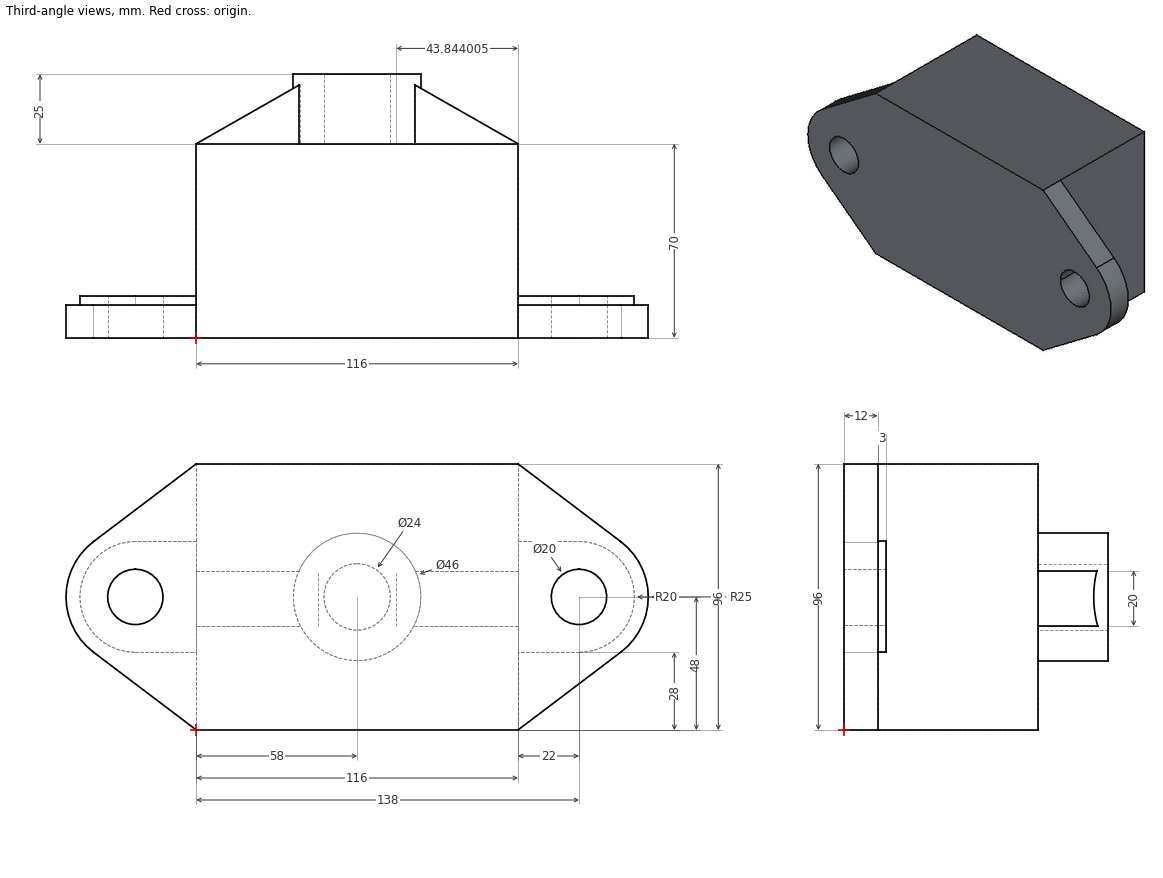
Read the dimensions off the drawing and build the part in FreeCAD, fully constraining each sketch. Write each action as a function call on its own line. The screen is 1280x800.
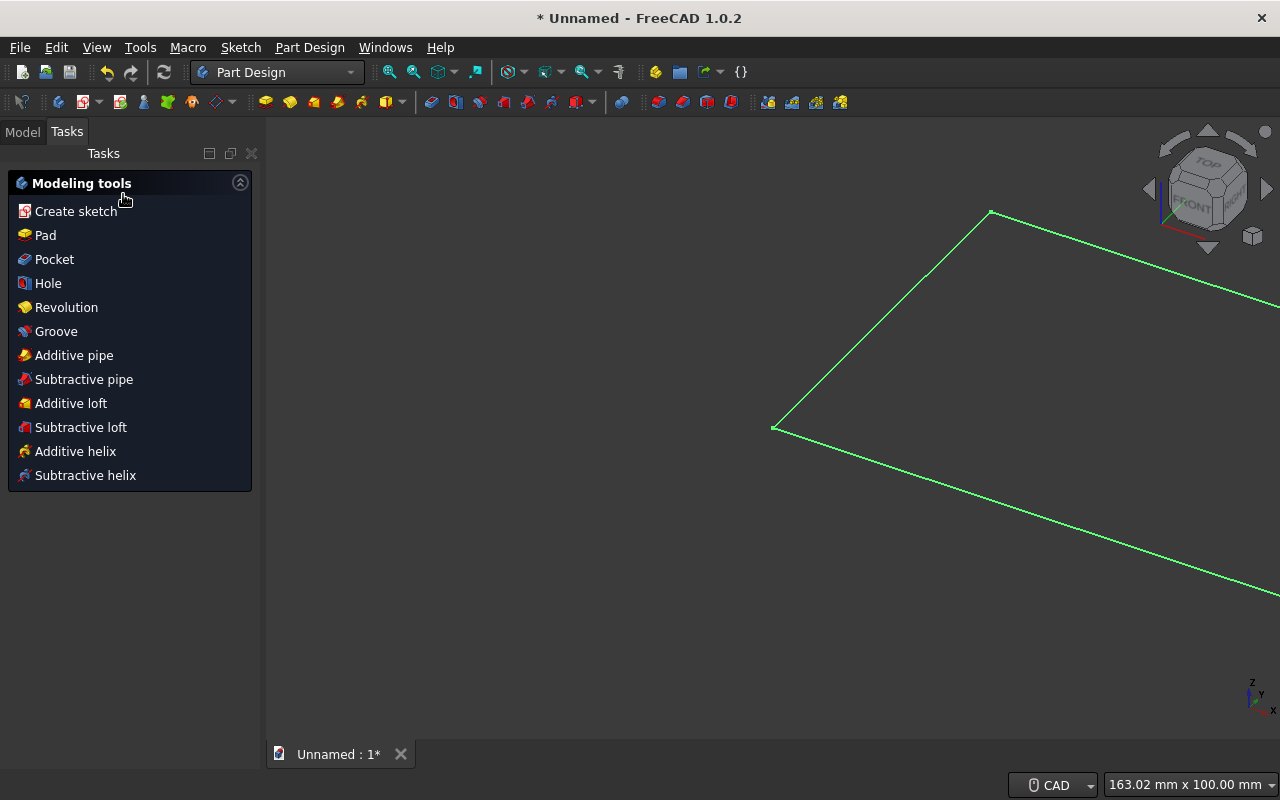
click(266, 102)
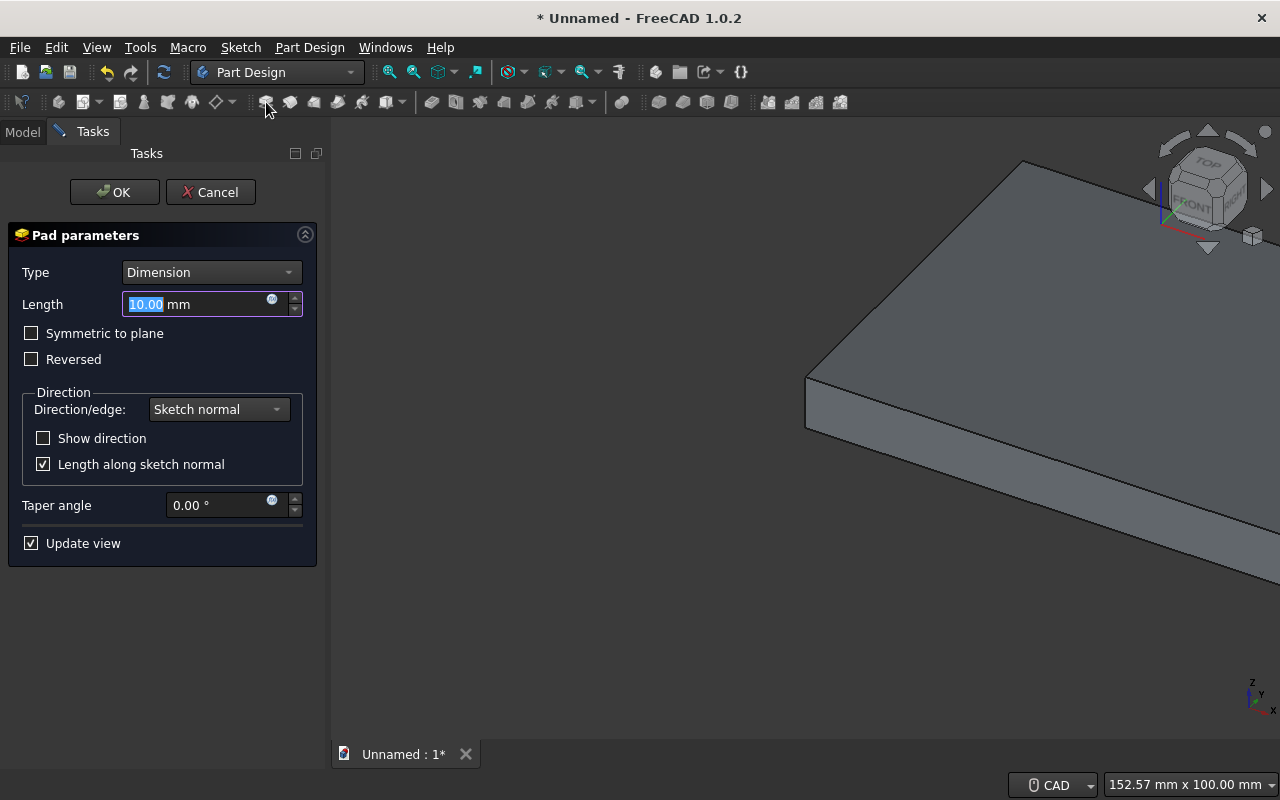
text(96)
key(Tab)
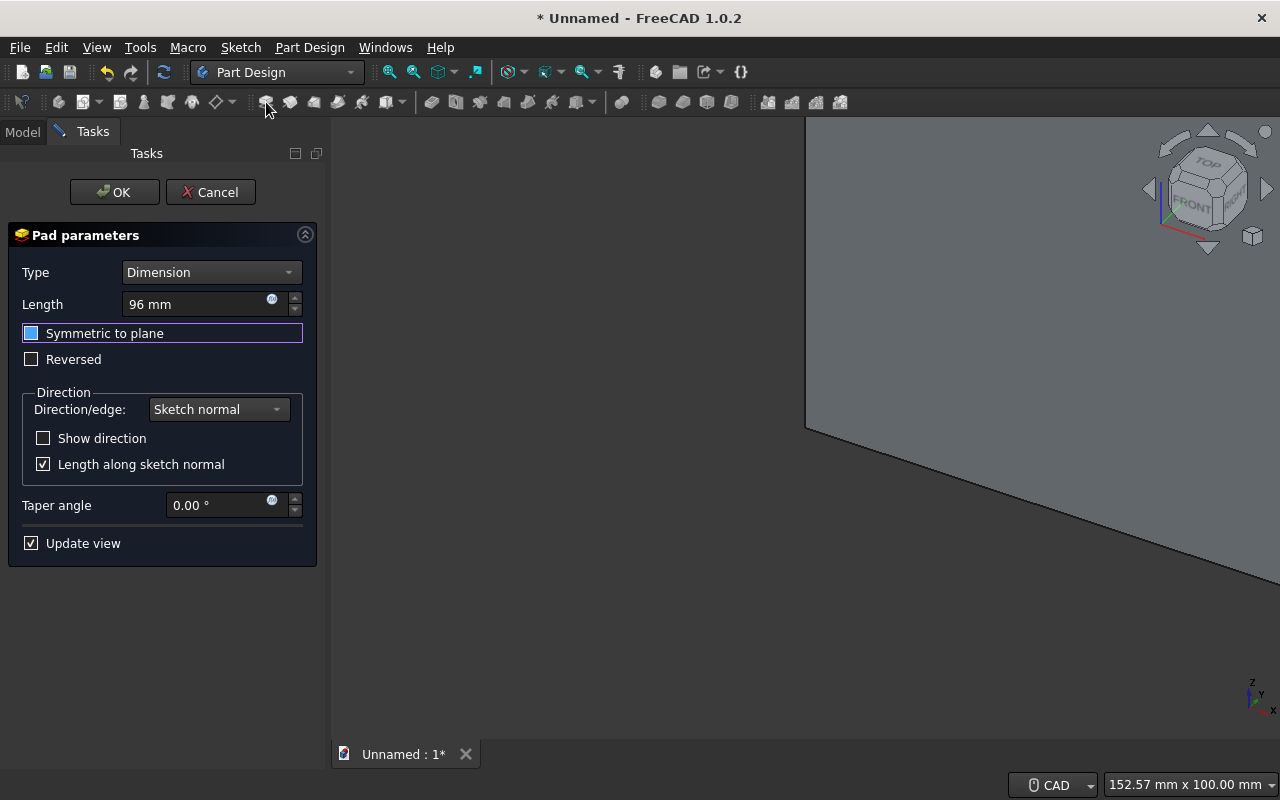
click(115, 192)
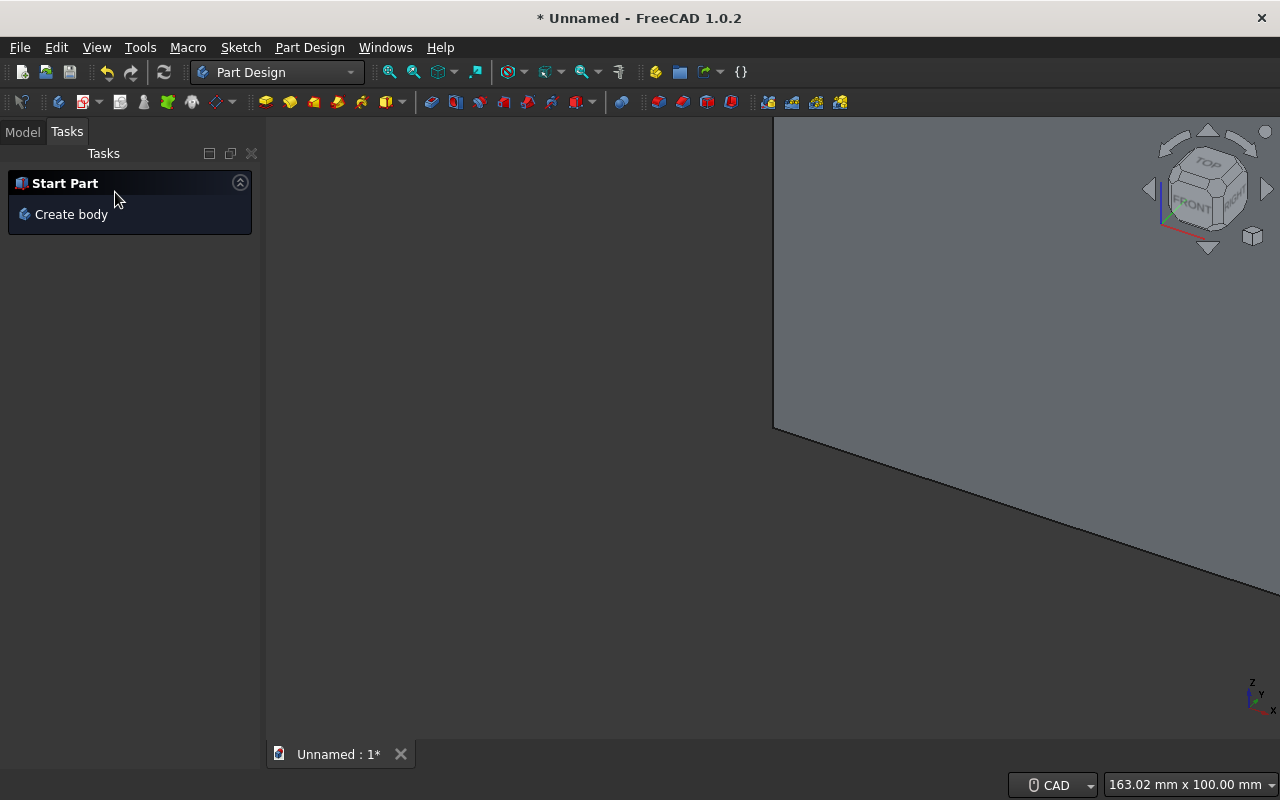
click(390, 72)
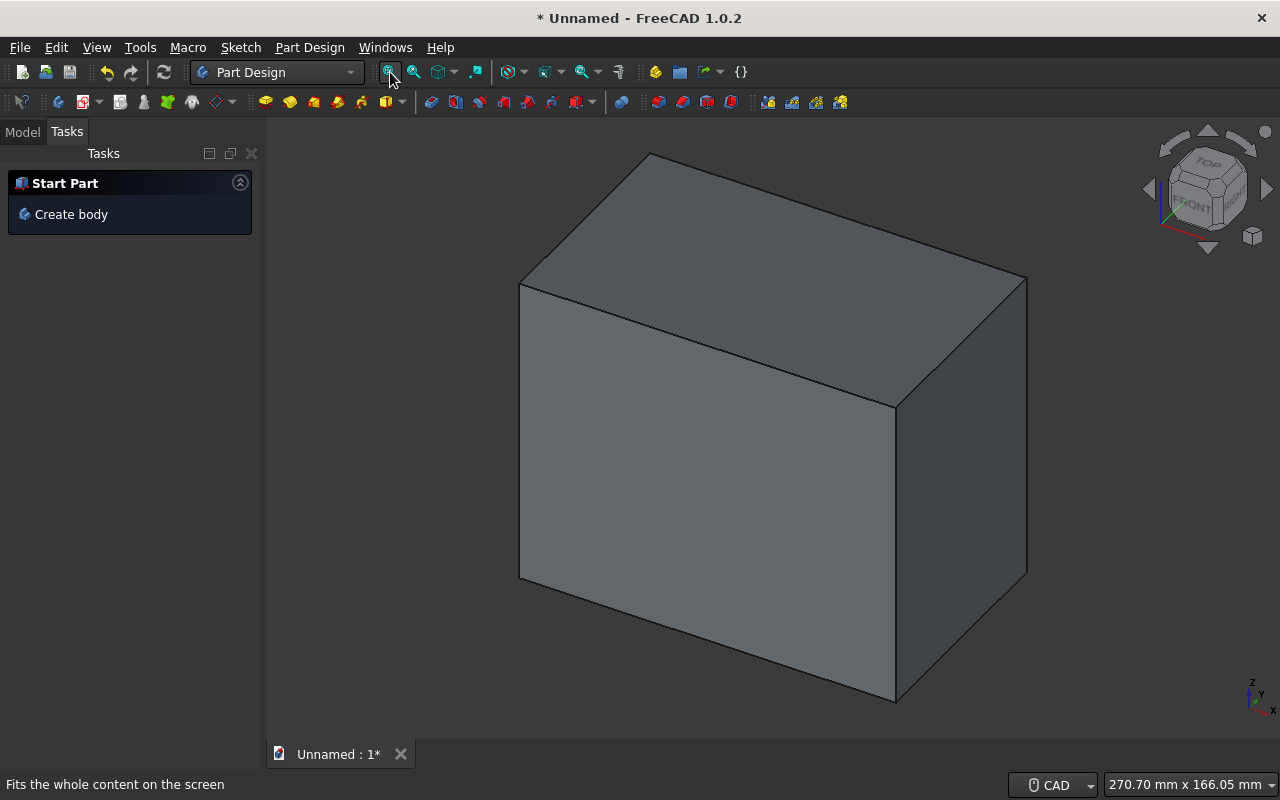
click(84, 102)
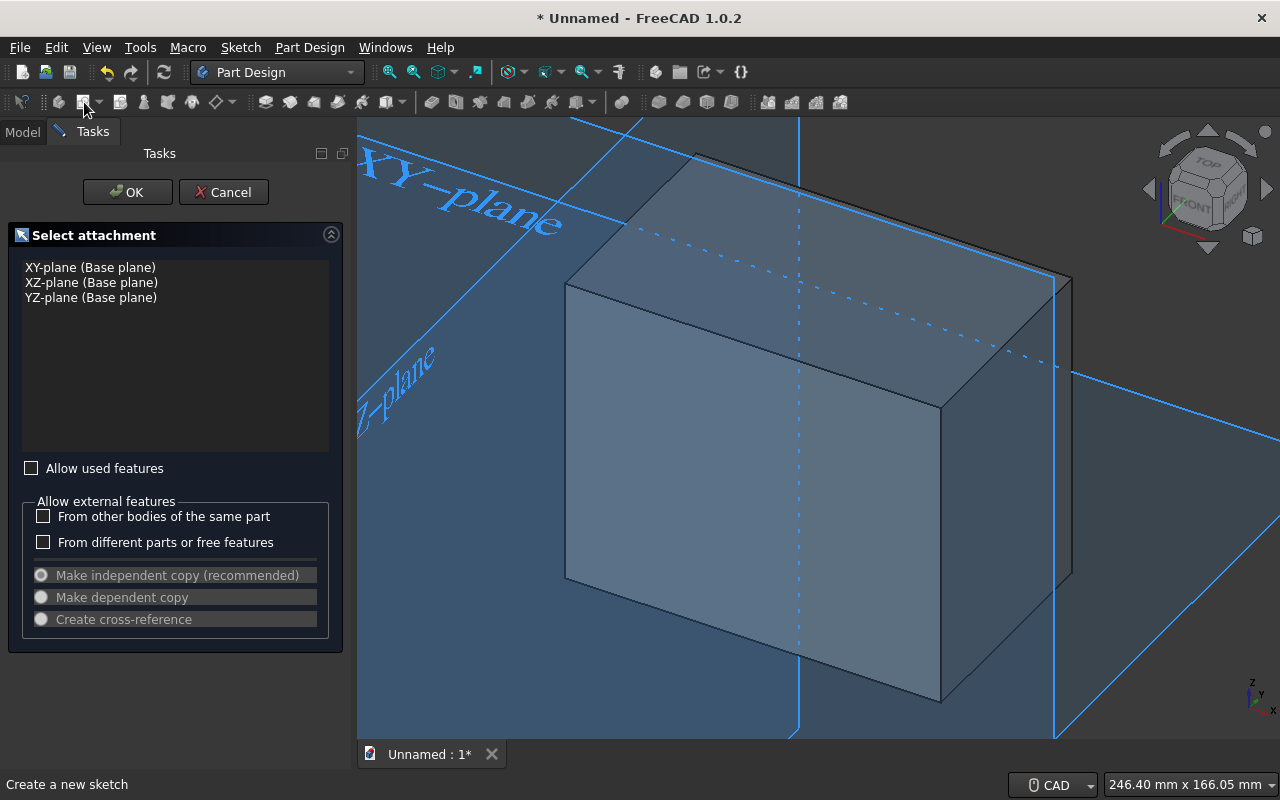
click(82, 282)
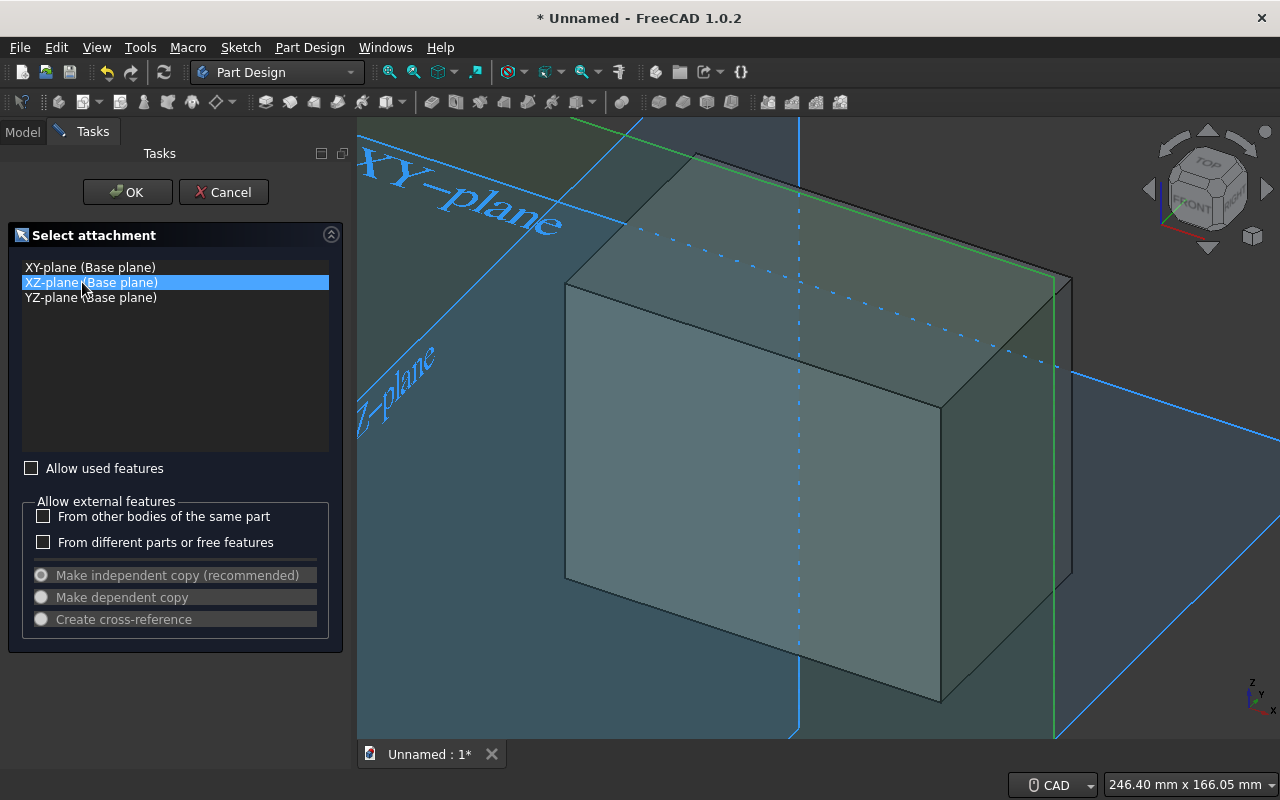
click(128, 192)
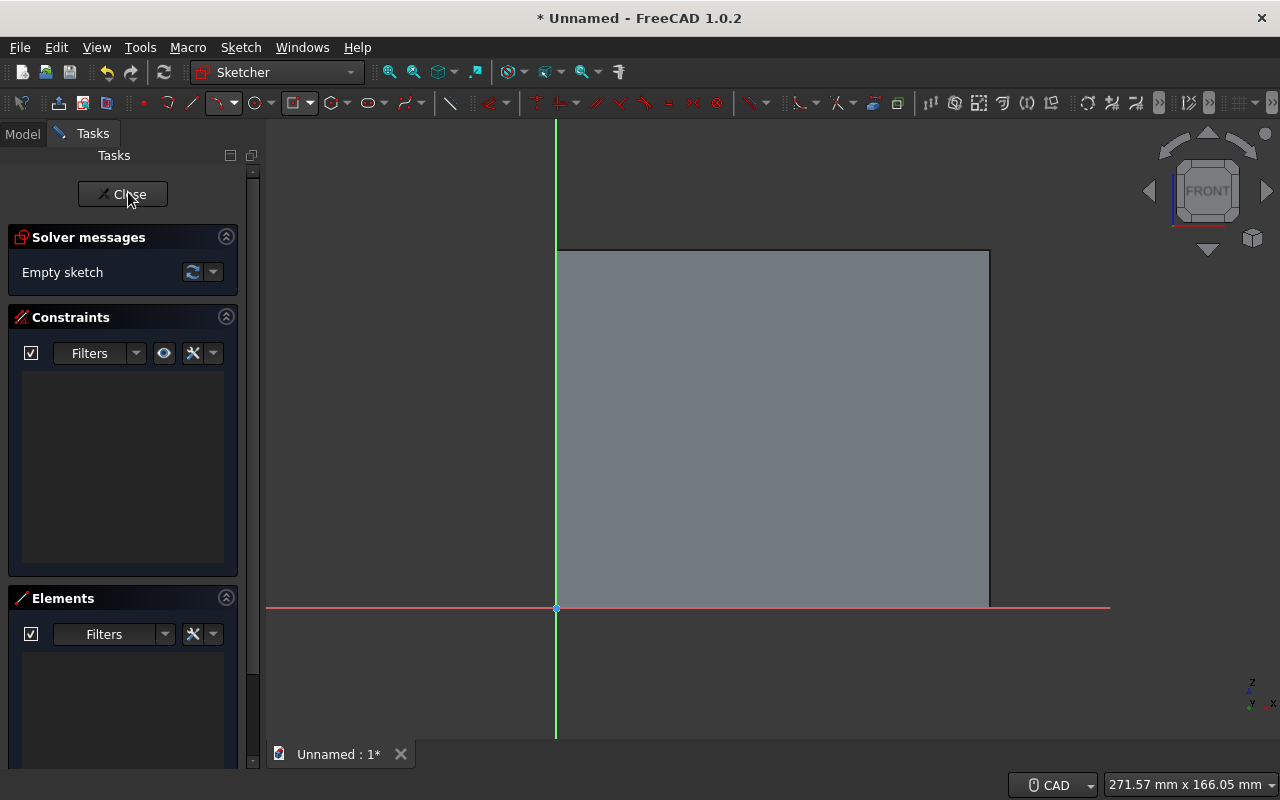
scroll(294, 429, down, 1)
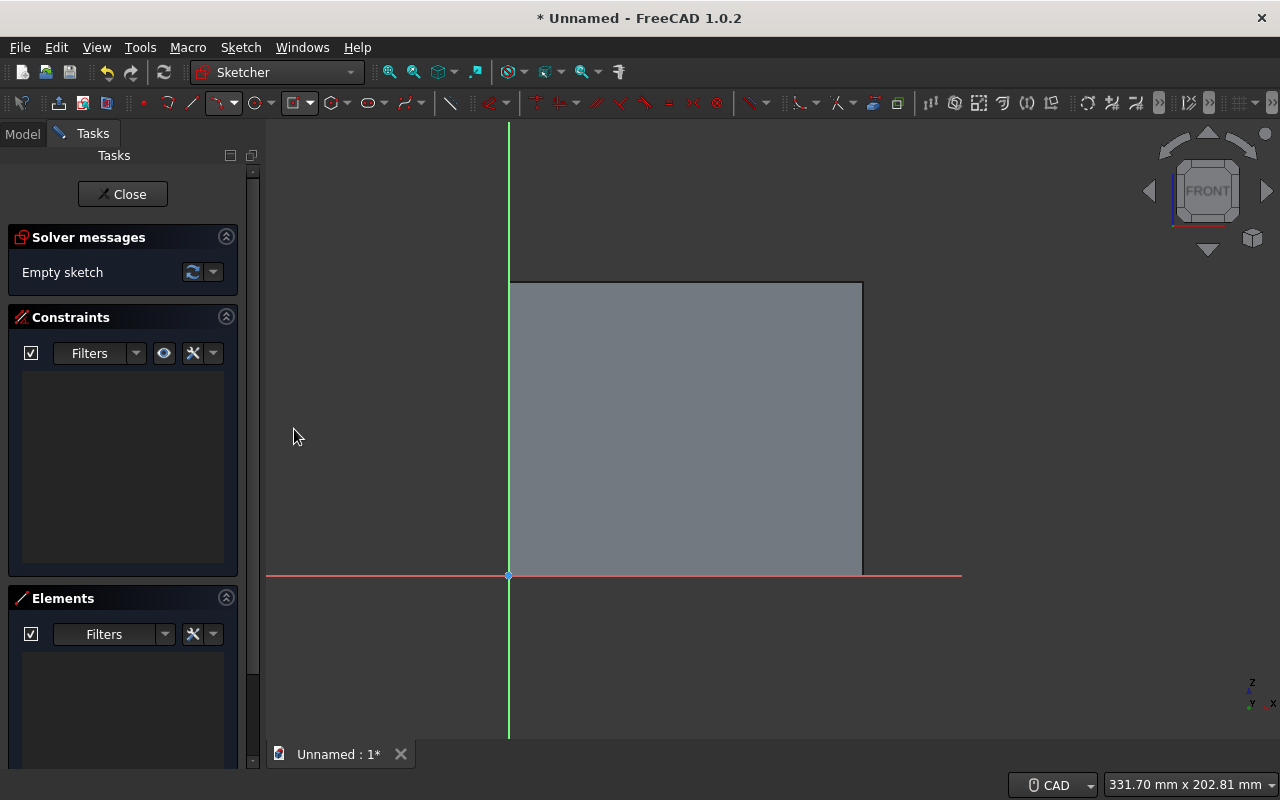
click(168, 104)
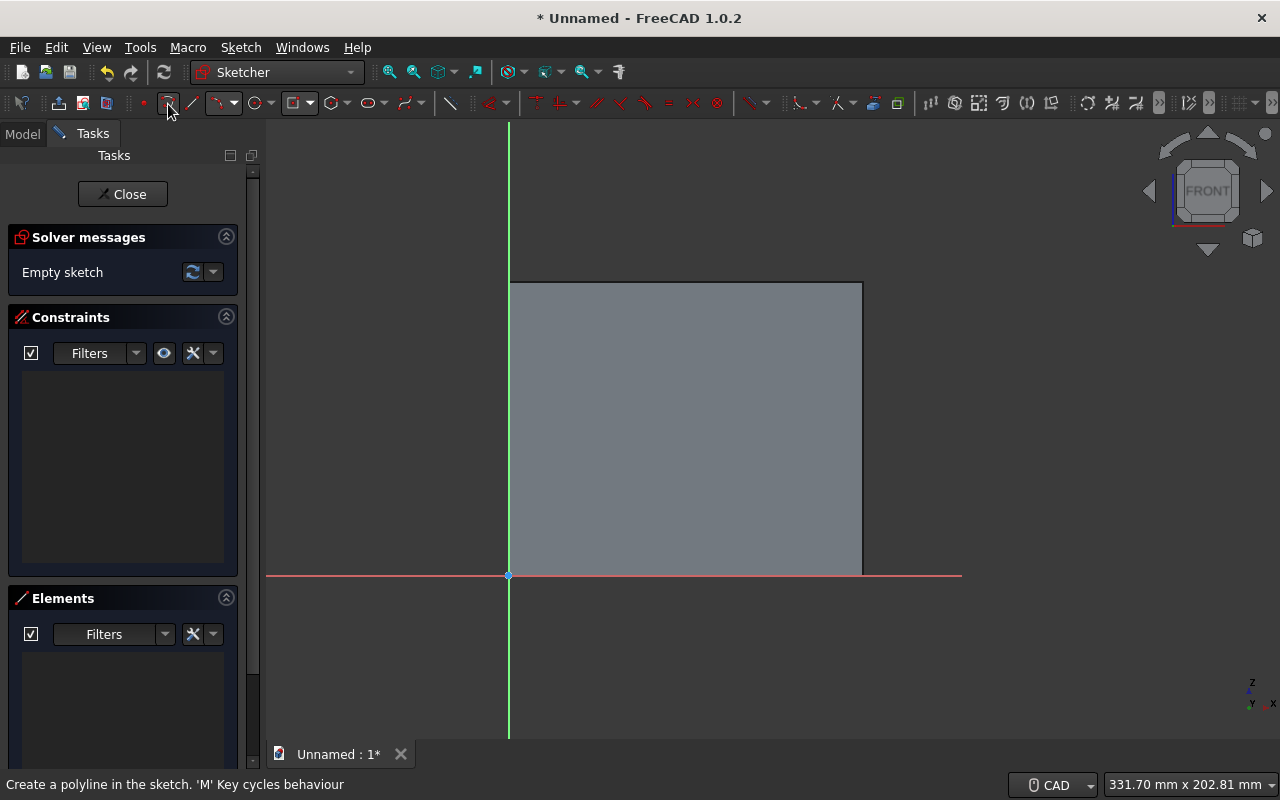
click(977, 490)
click(863, 576)
click(863, 282)
click(977, 368)
right_click(977, 368)